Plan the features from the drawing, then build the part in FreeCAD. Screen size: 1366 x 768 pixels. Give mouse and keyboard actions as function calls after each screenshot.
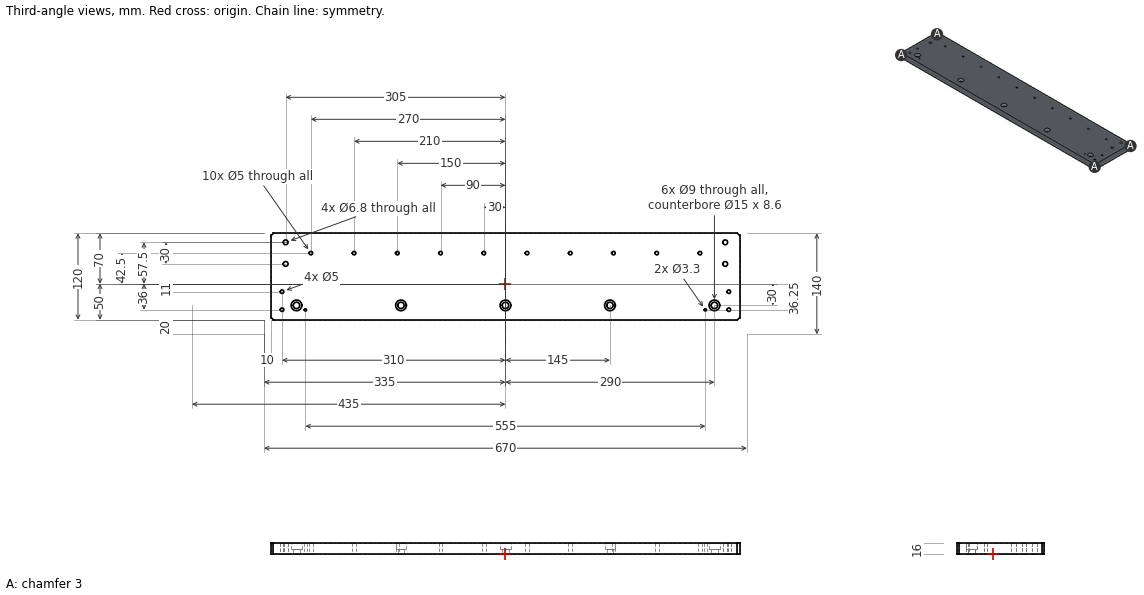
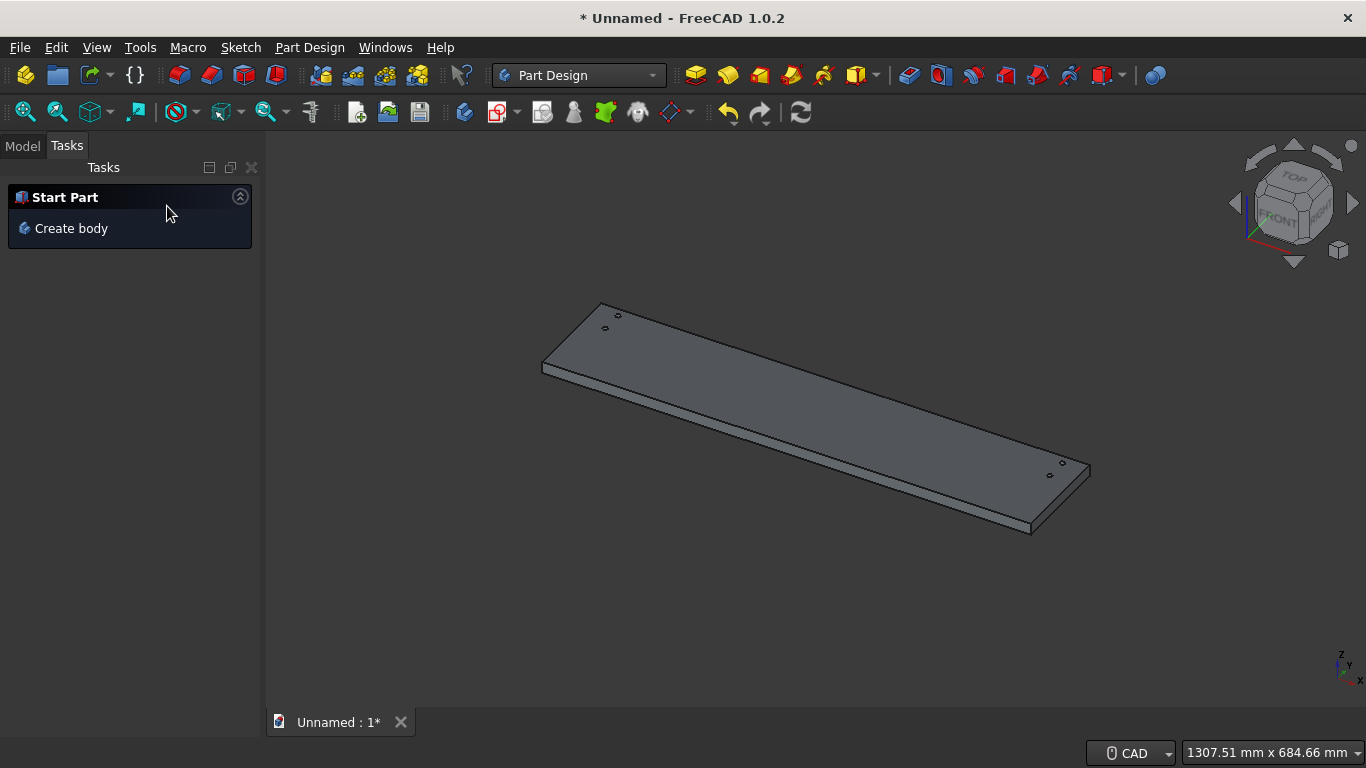
click(955, 459)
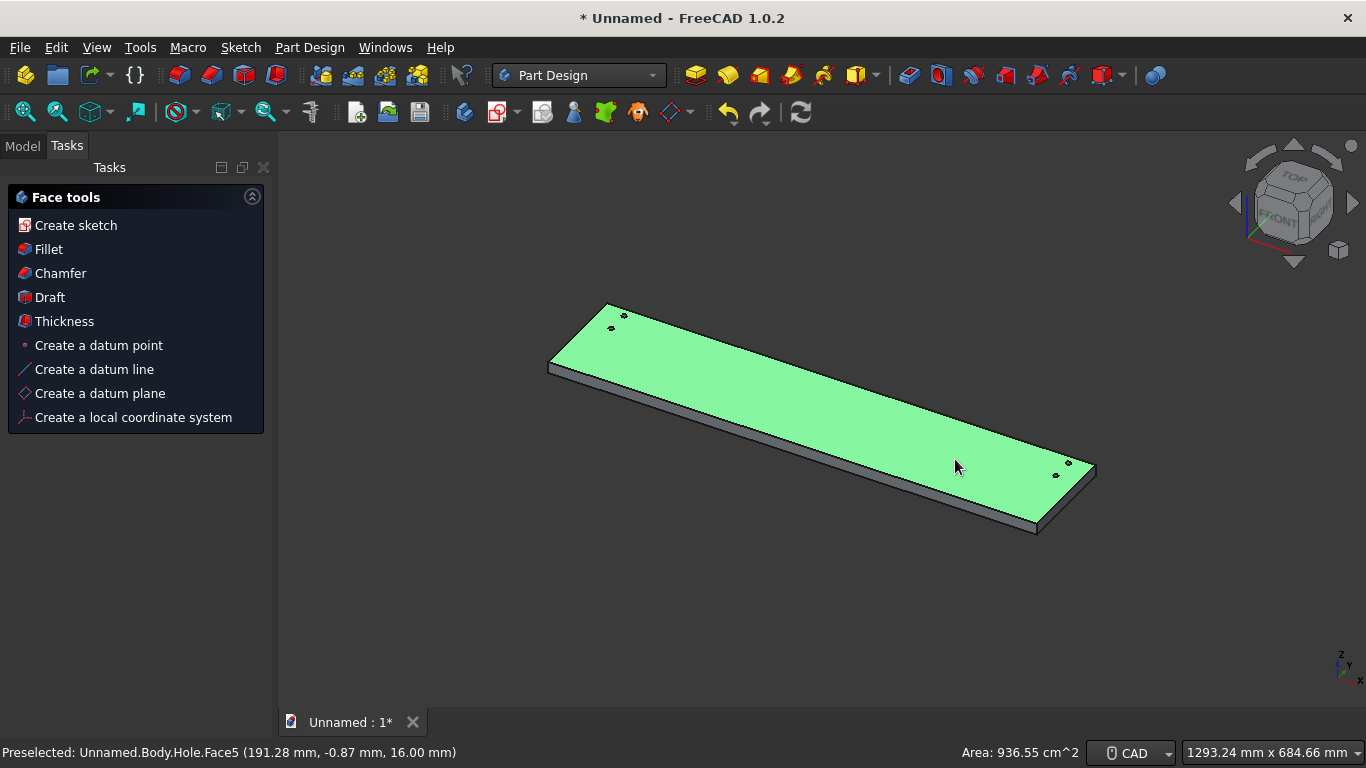
click(498, 112)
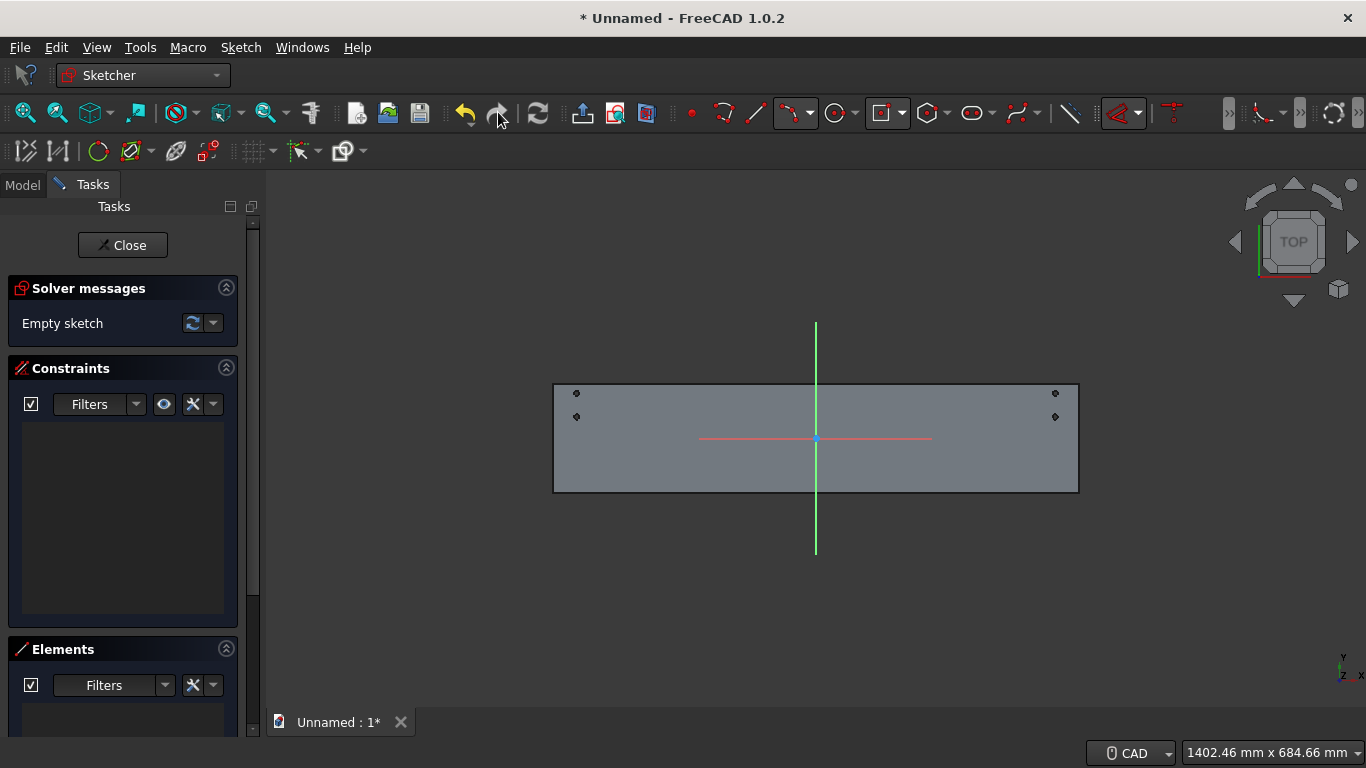
scroll(955, 385, up, 2)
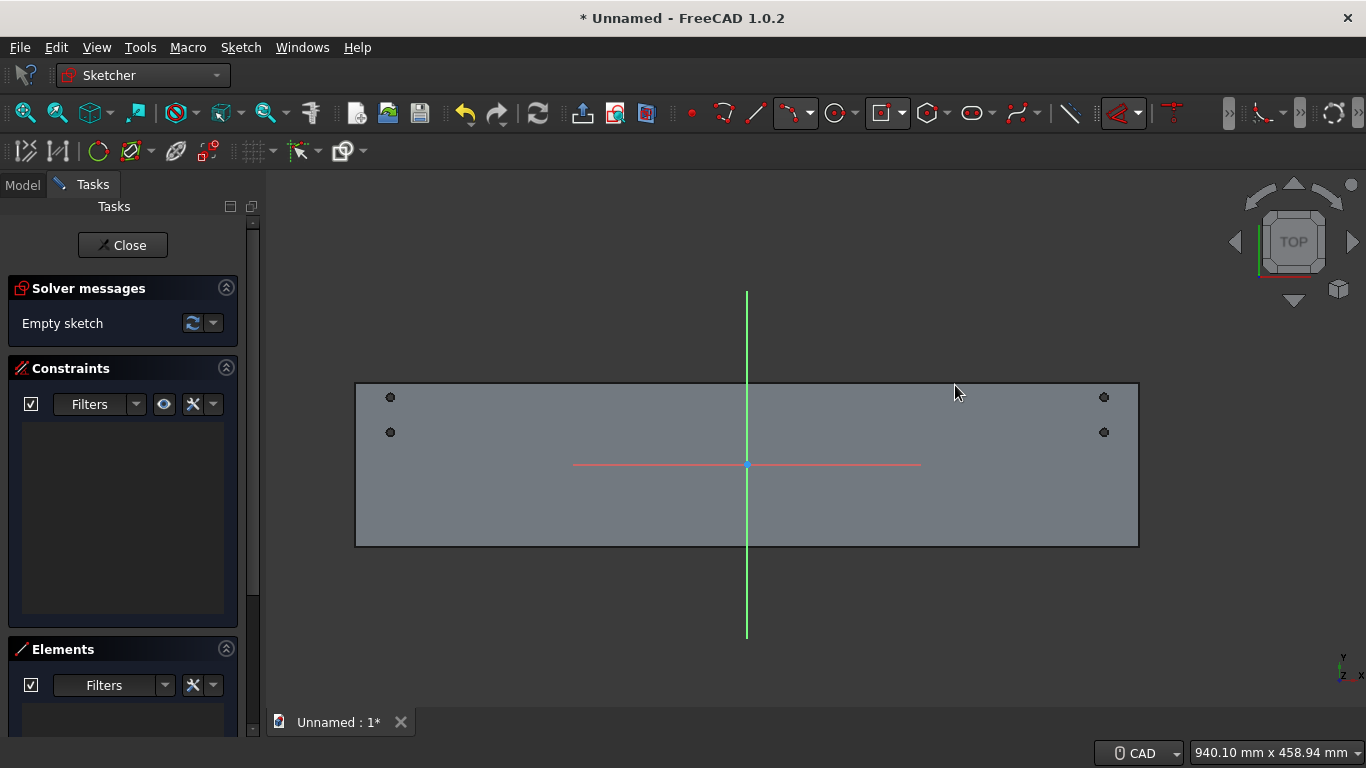
click(836, 114)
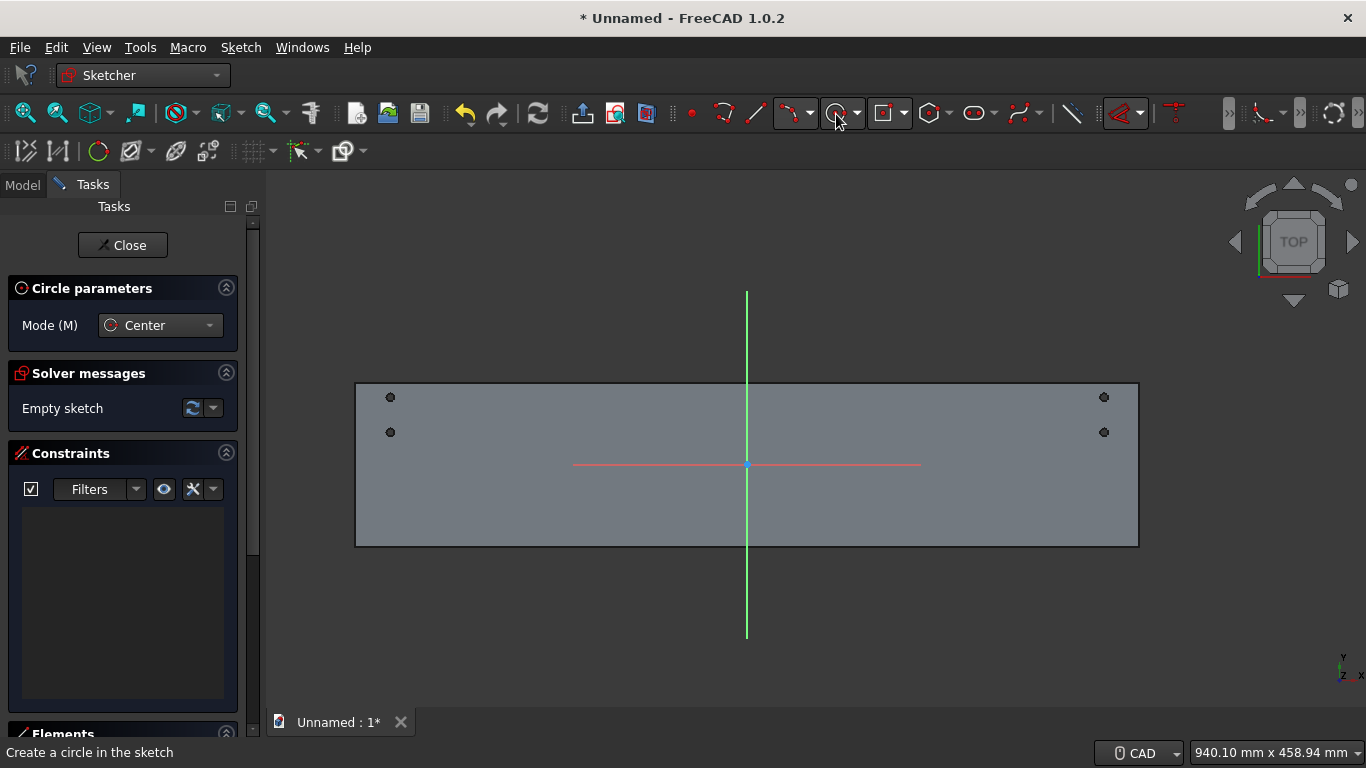
scroll(431, 415, up, 11)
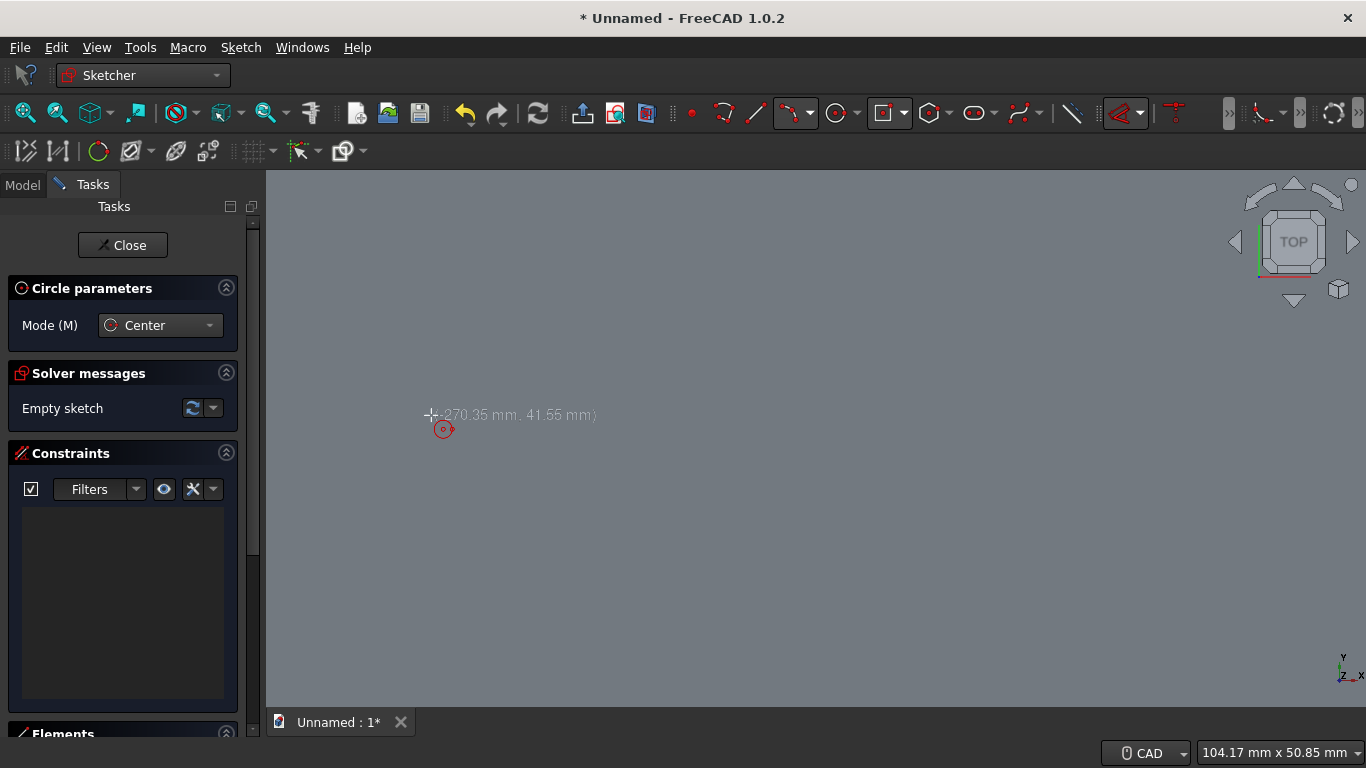
scroll(431, 416, down, 11)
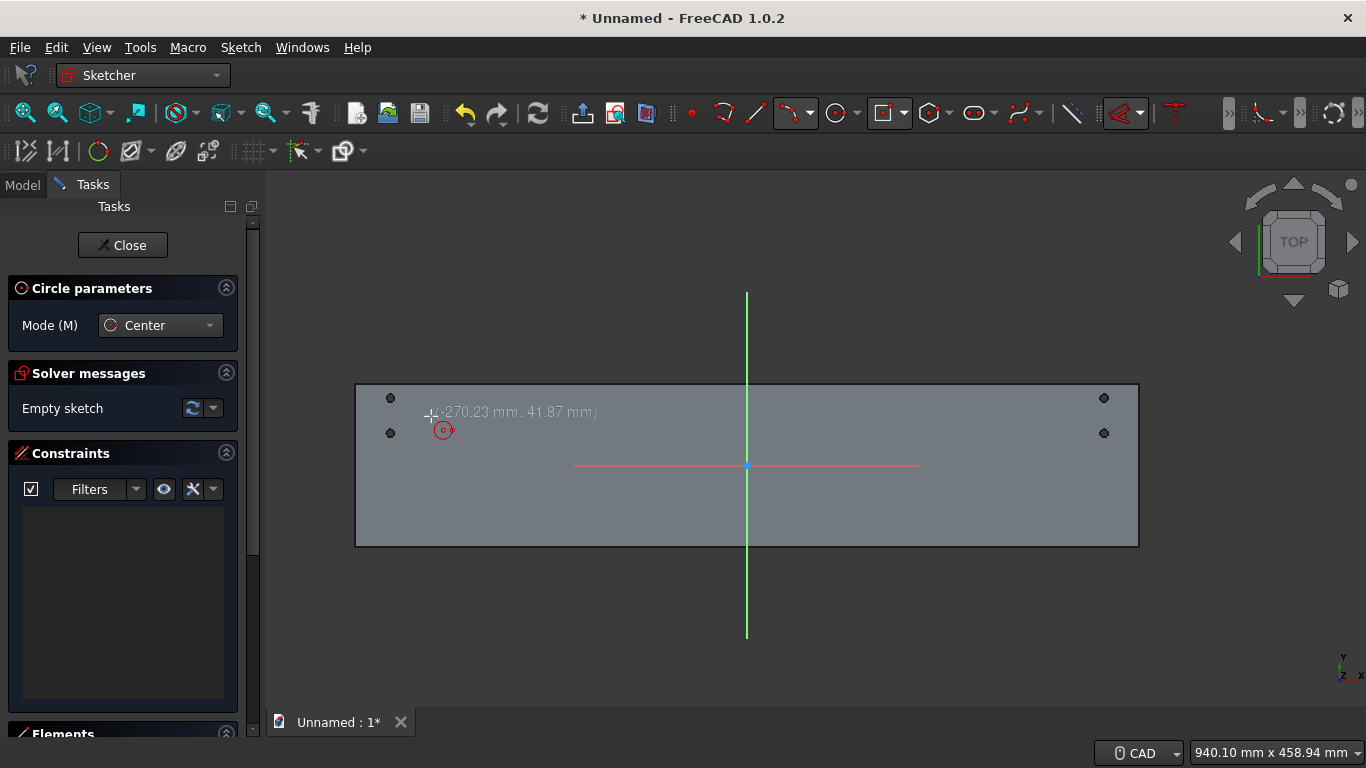
click(431, 416)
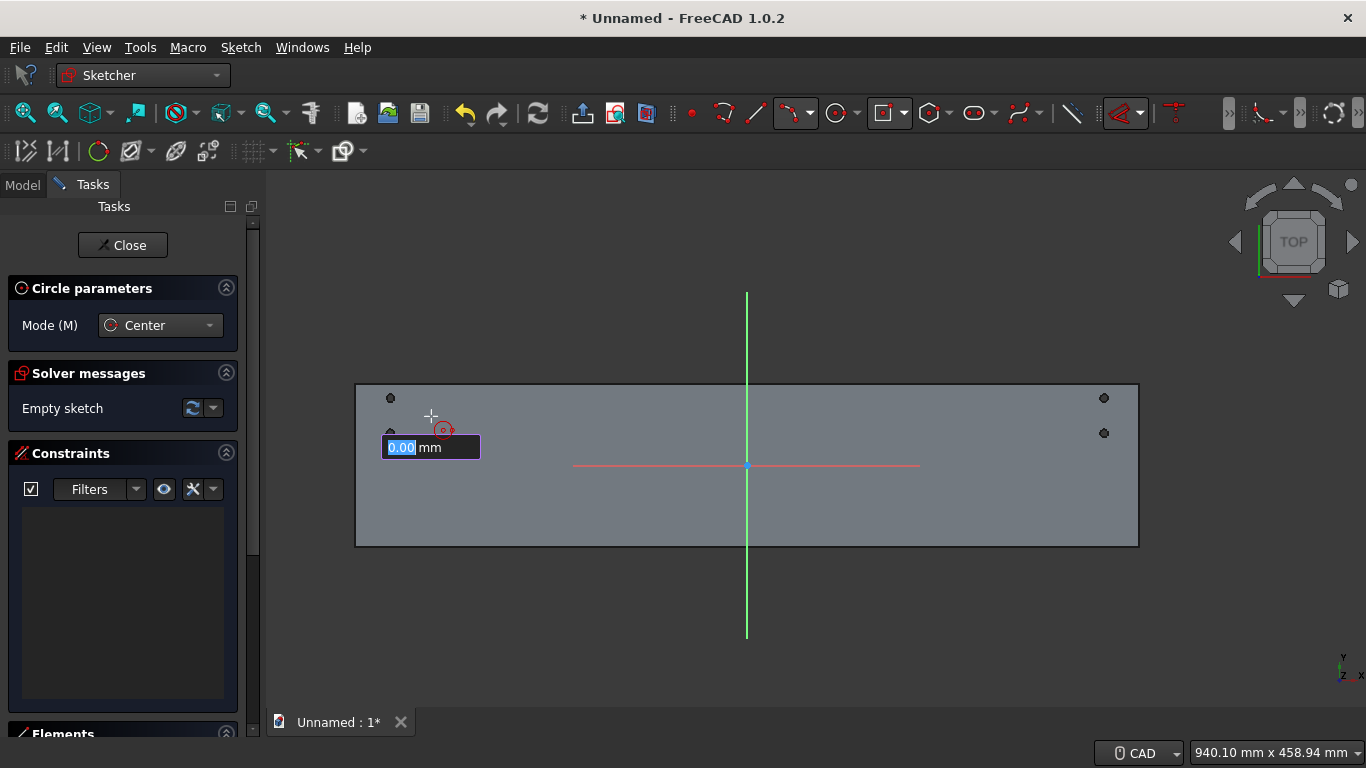
scroll(433, 414, up, 9)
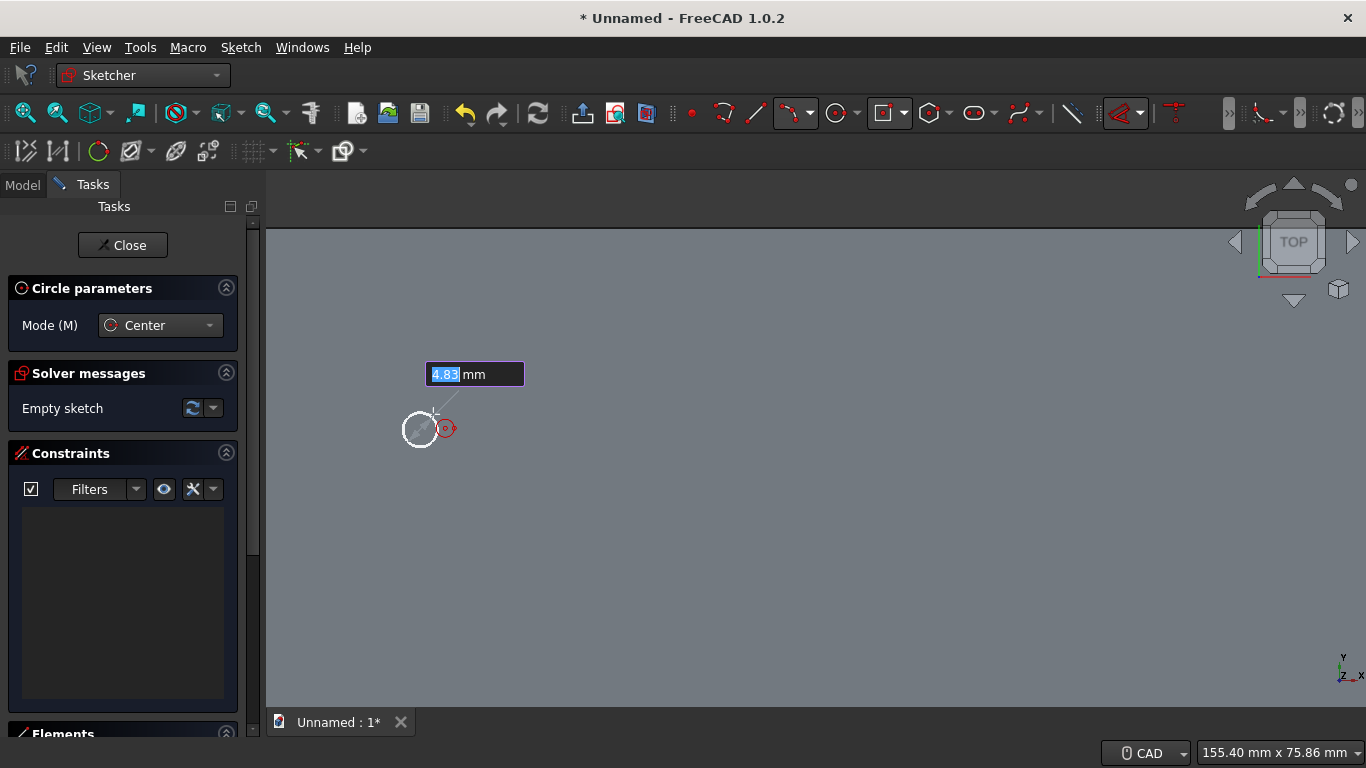
click(435, 410)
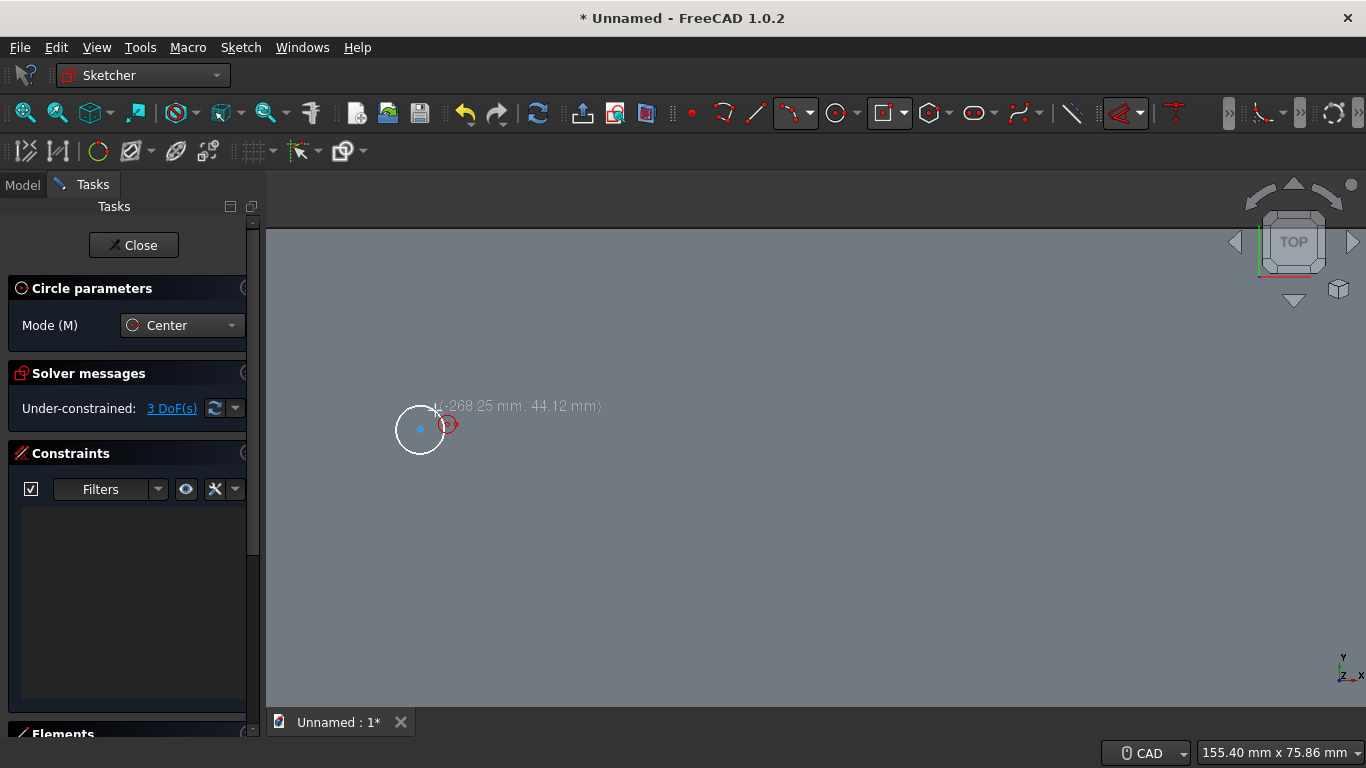
scroll(847, 422, up, 2)